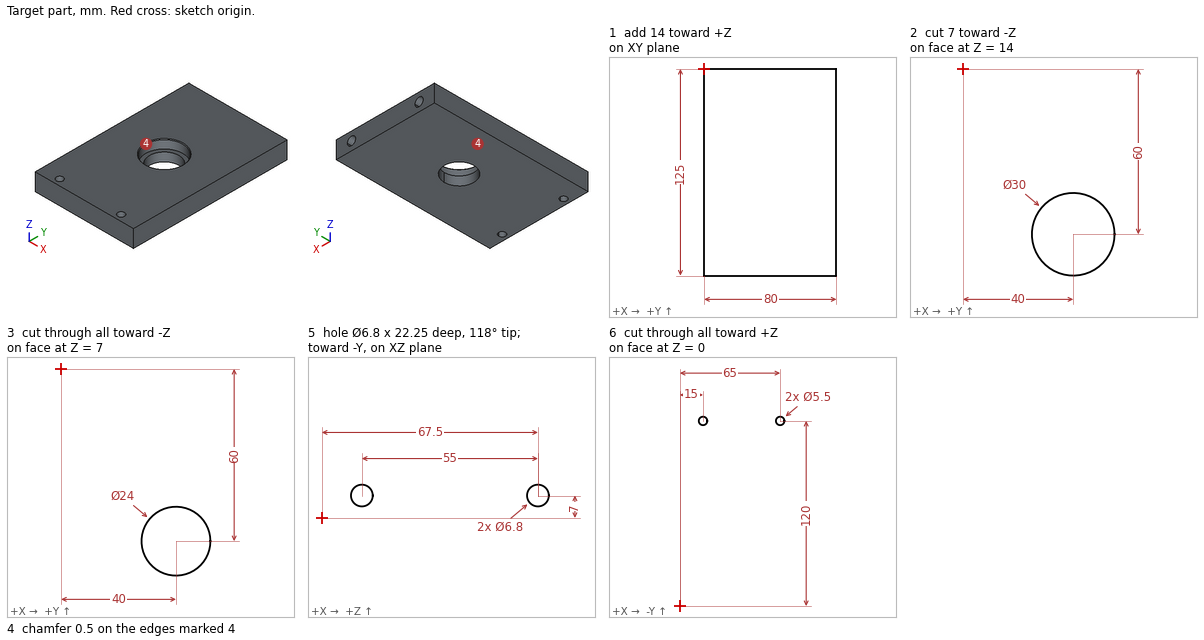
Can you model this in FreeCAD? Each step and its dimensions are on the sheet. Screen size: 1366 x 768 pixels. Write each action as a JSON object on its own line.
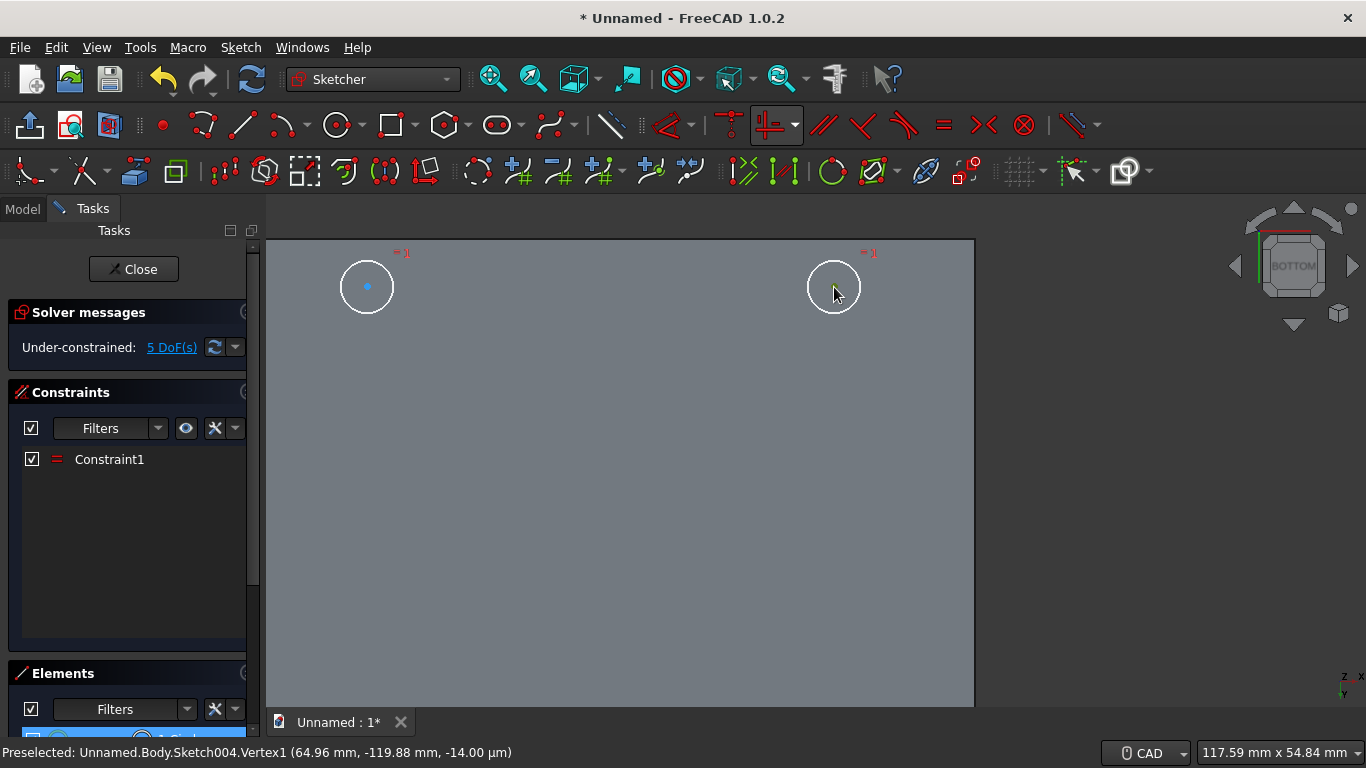
{"action": "left_click", "coordinate": [367, 287]}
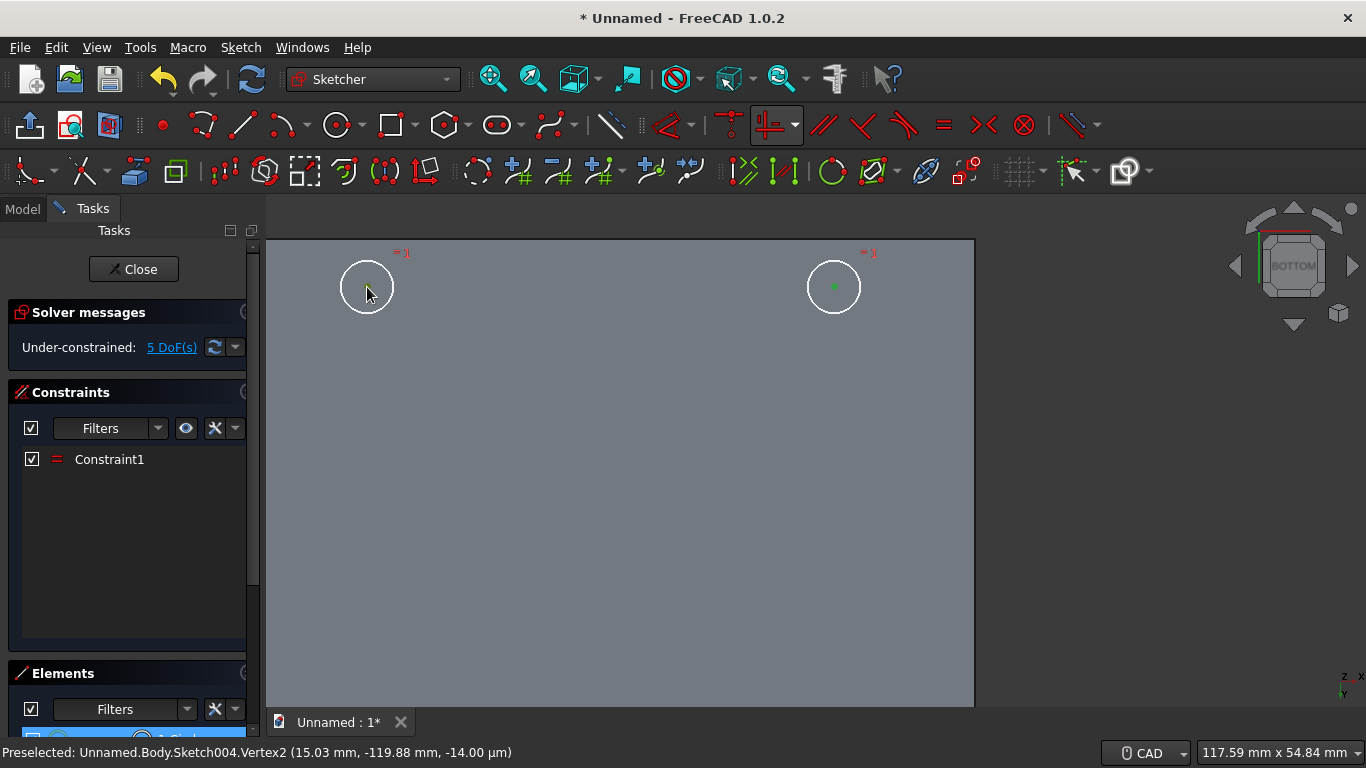
{"action": "key", "text": "h"}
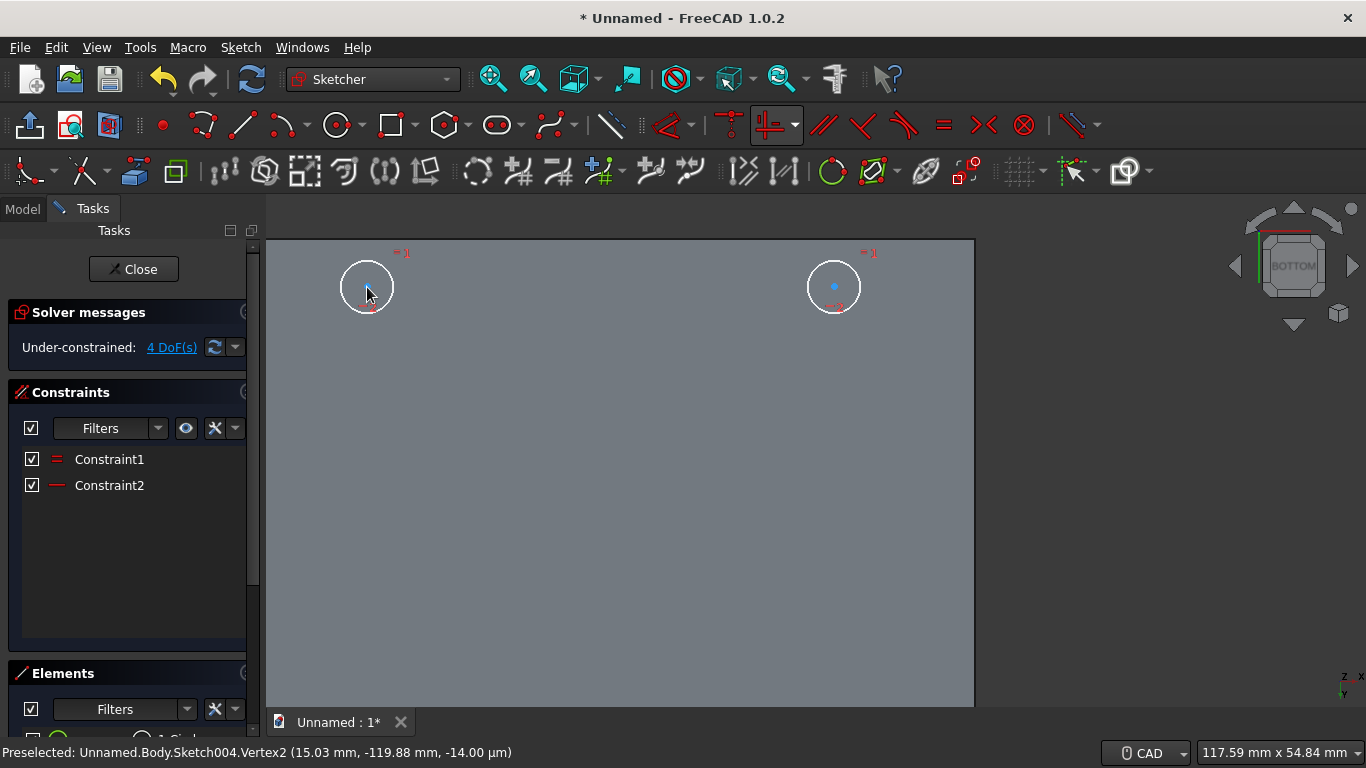
{"action": "left_click", "coordinate": [666, 126]}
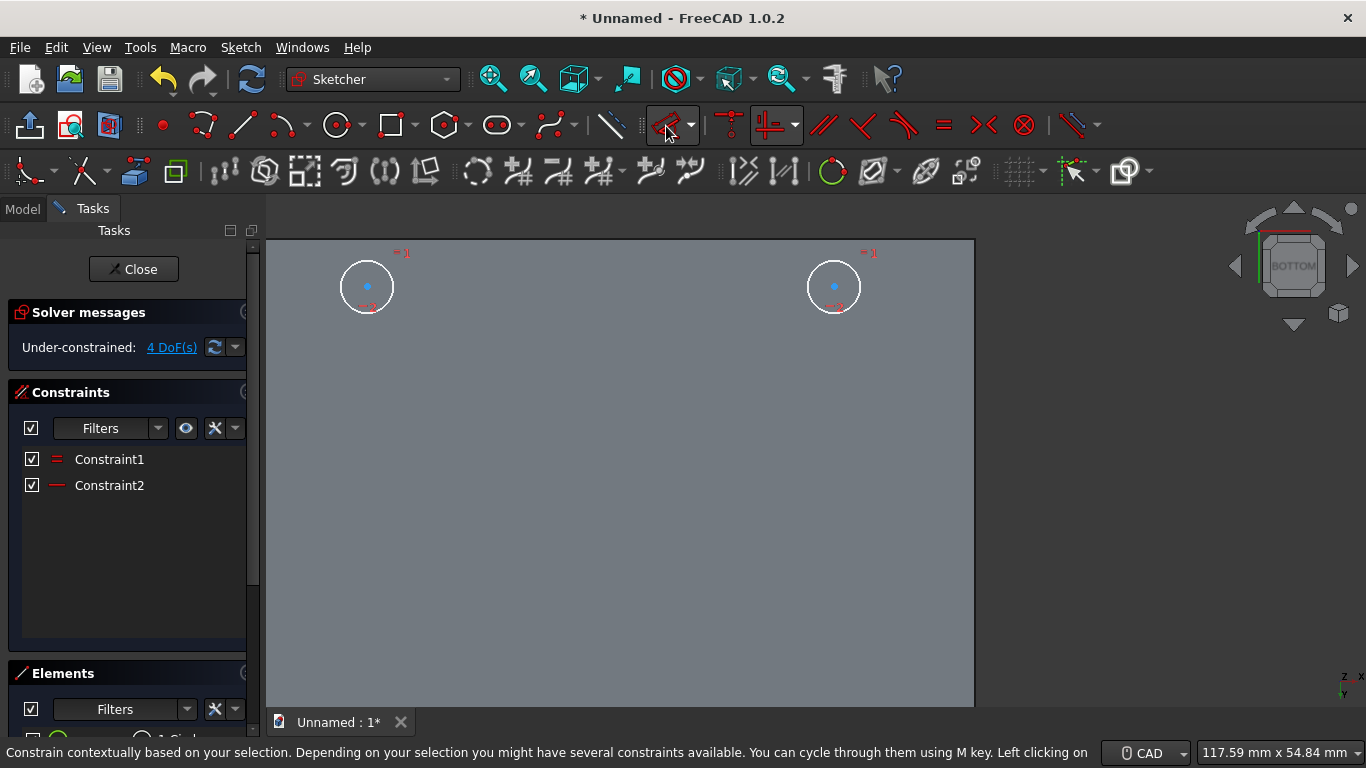
{"action": "left_click", "coordinate": [852, 268]}
{"action": "left_click", "coordinate": [874, 245]}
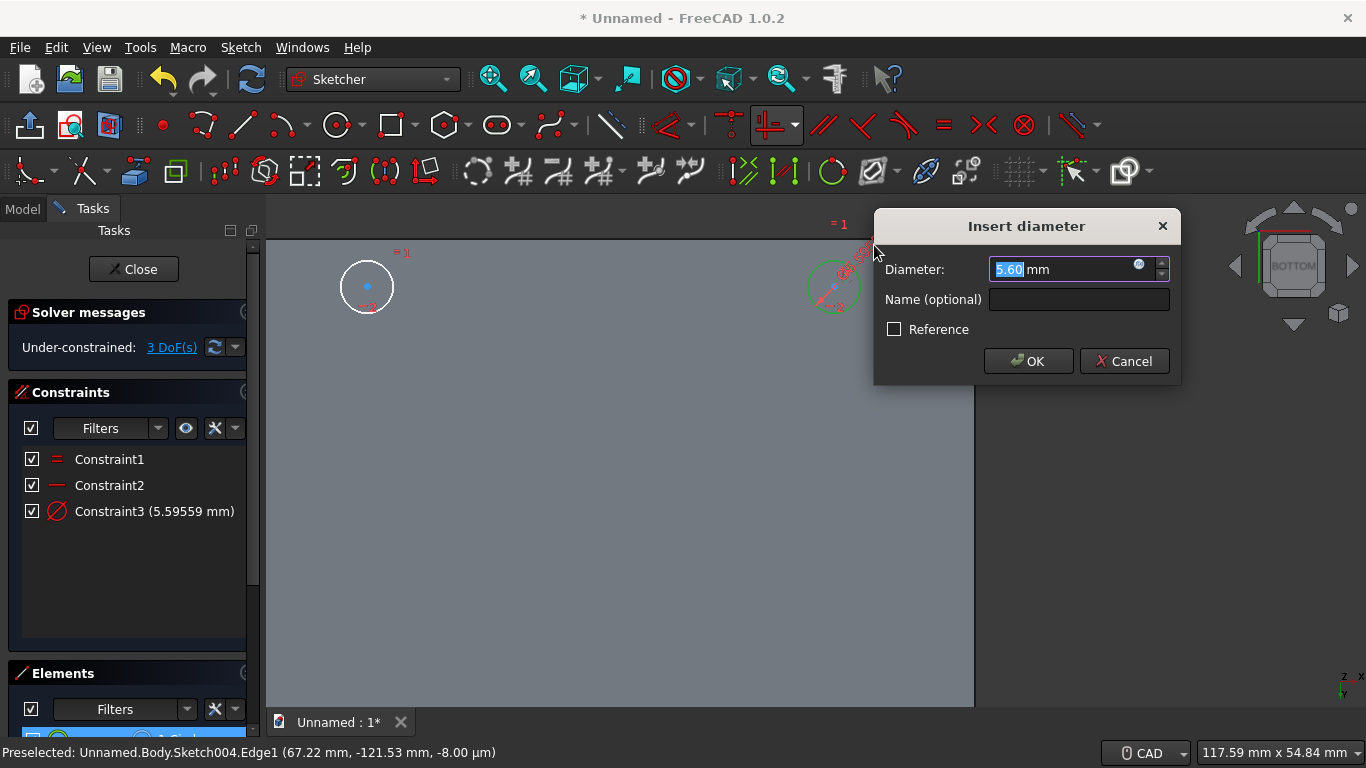
{"action": "type", "text": "5.5"}
{"action": "key", "text": "Return"}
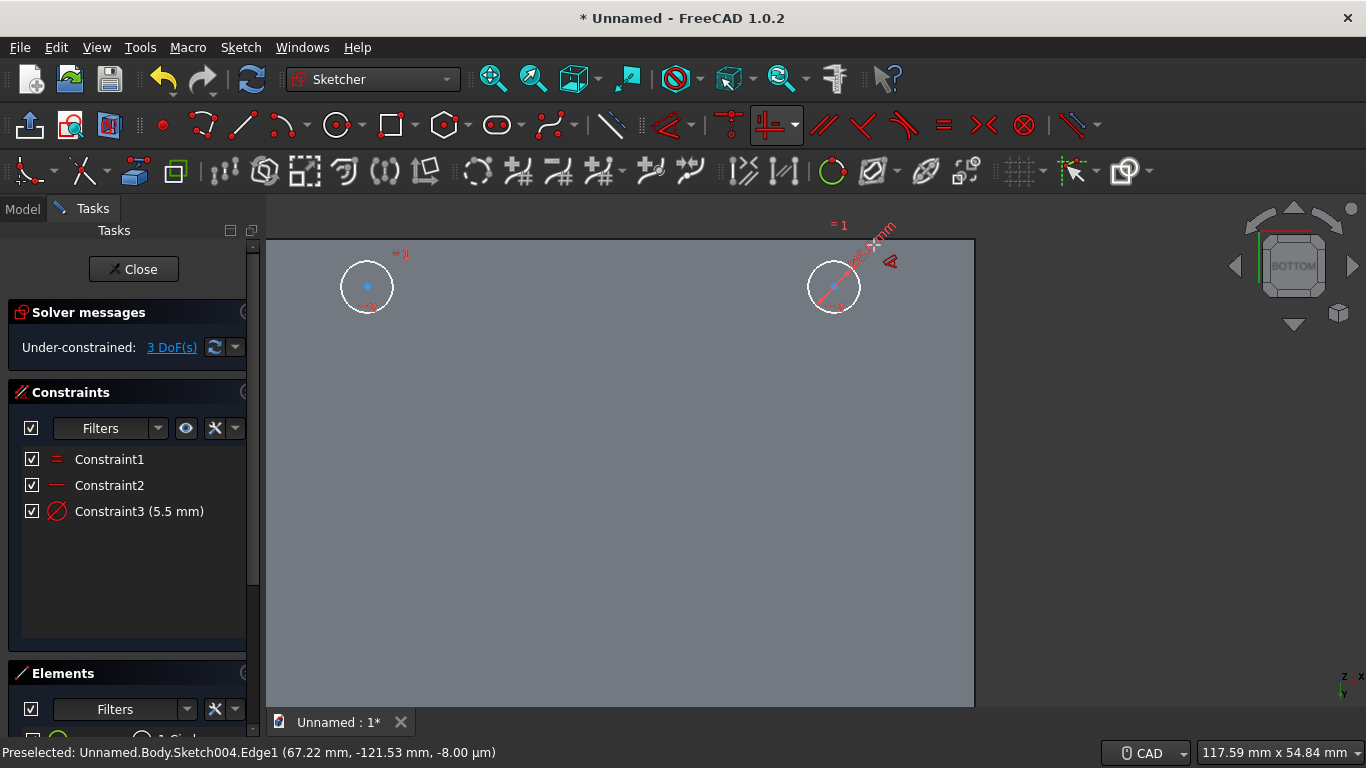
{"action": "left_click", "coordinate": [834, 287]}
{"action": "left_click", "coordinate": [564, 253]}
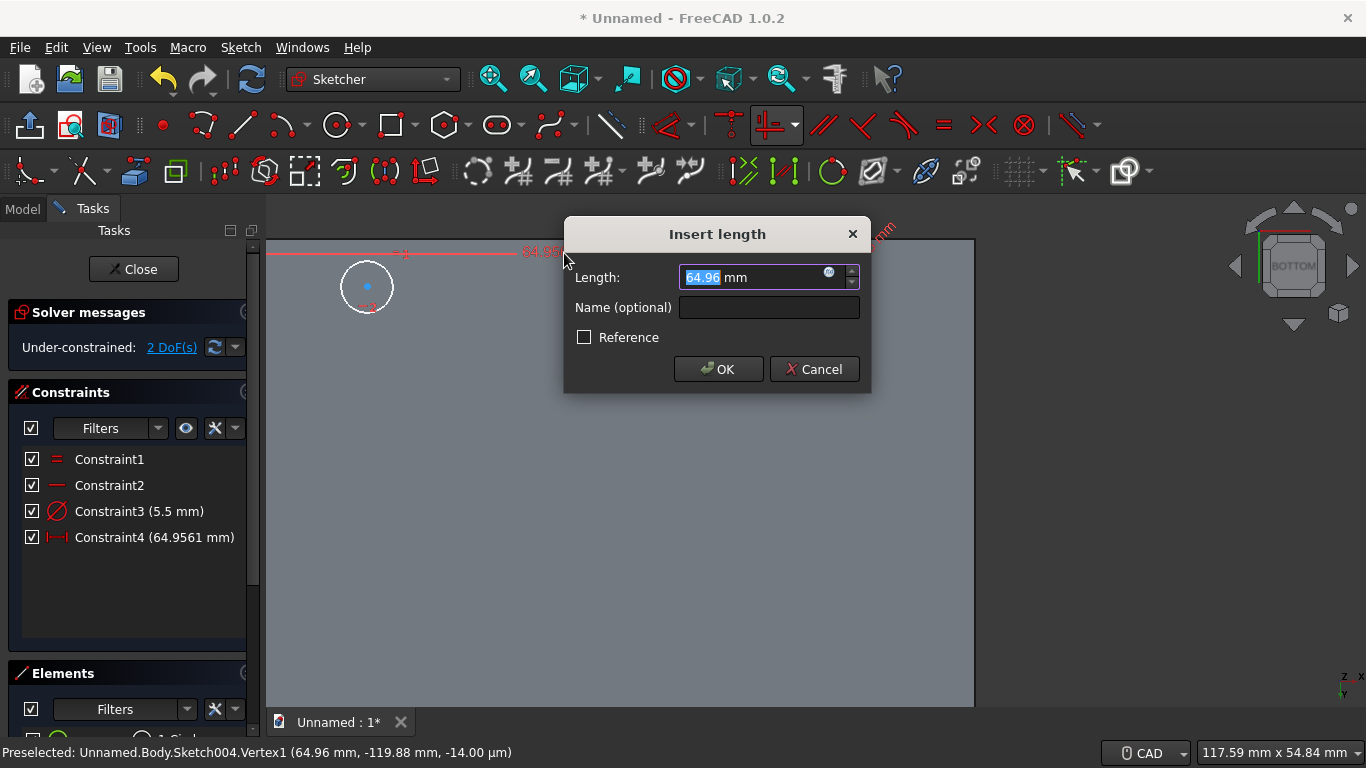
{"action": "type", "text": "65"}
{"action": "key", "text": "Return"}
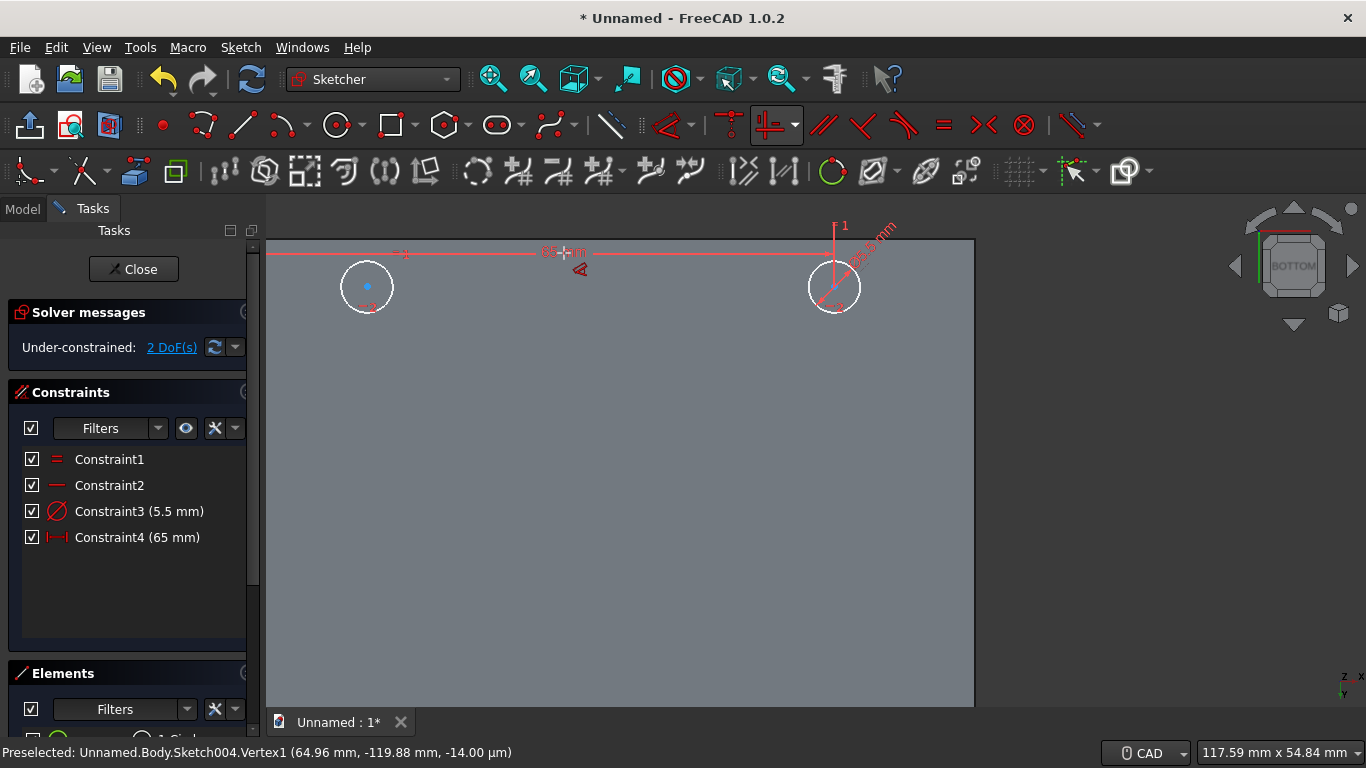
{"action": "left_click", "coordinate": [367, 287]}
{"action": "left_click", "coordinate": [331, 253]}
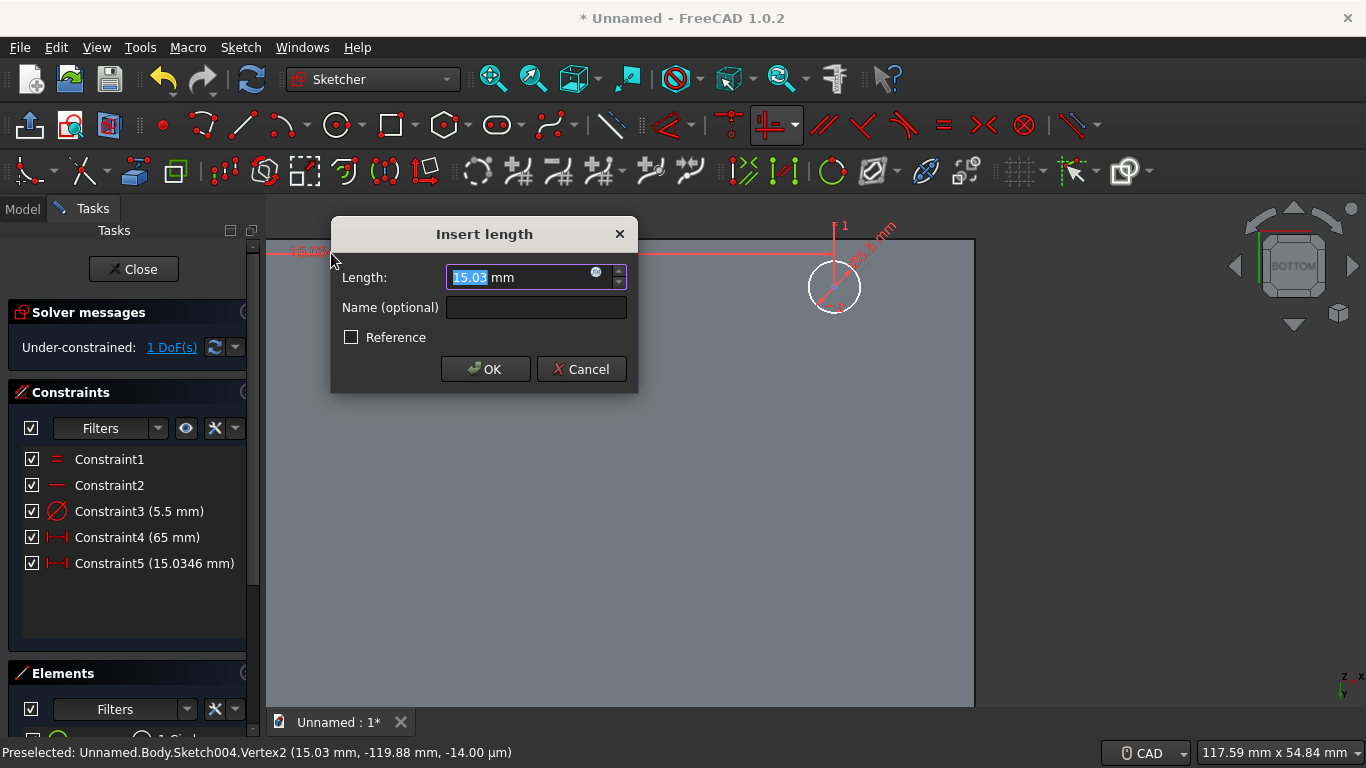
{"action": "type", "text": "15"}
{"action": "key", "text": "Return"}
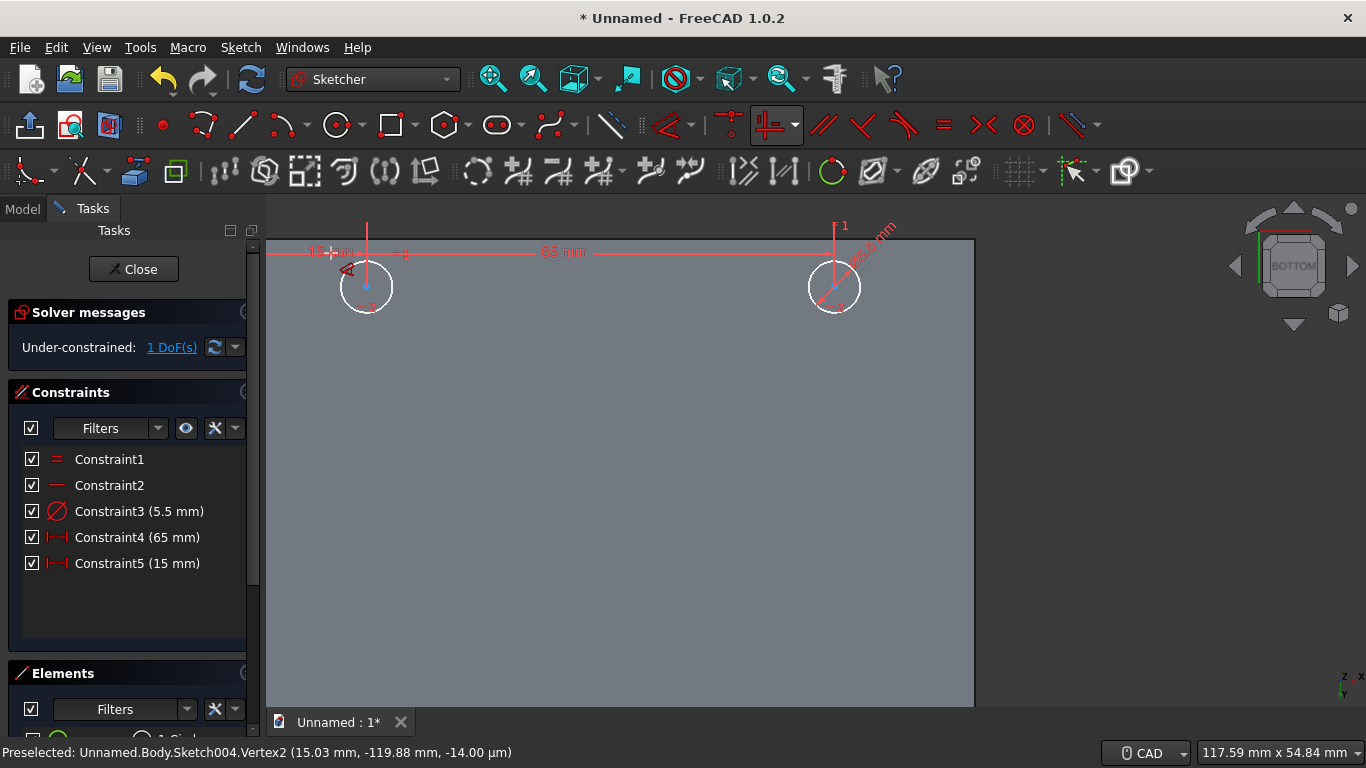
{"action": "left_click", "coordinate": [834, 287]}
{"action": "left_click", "coordinate": [868, 483]}